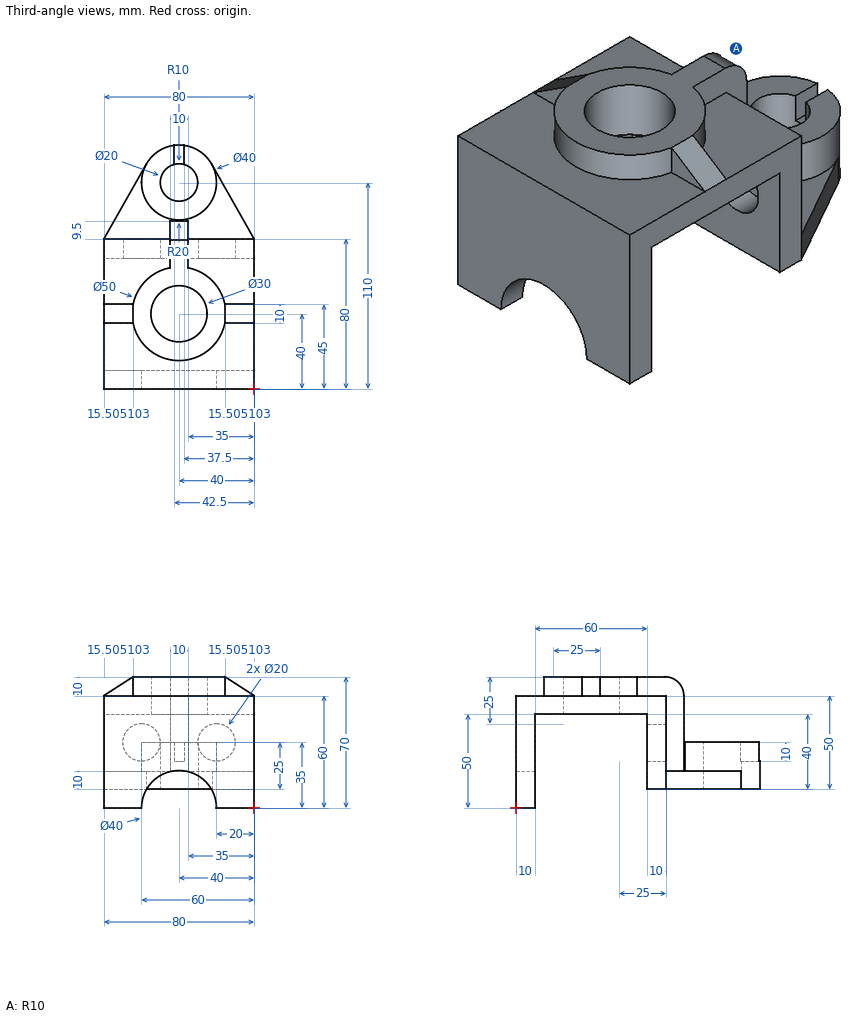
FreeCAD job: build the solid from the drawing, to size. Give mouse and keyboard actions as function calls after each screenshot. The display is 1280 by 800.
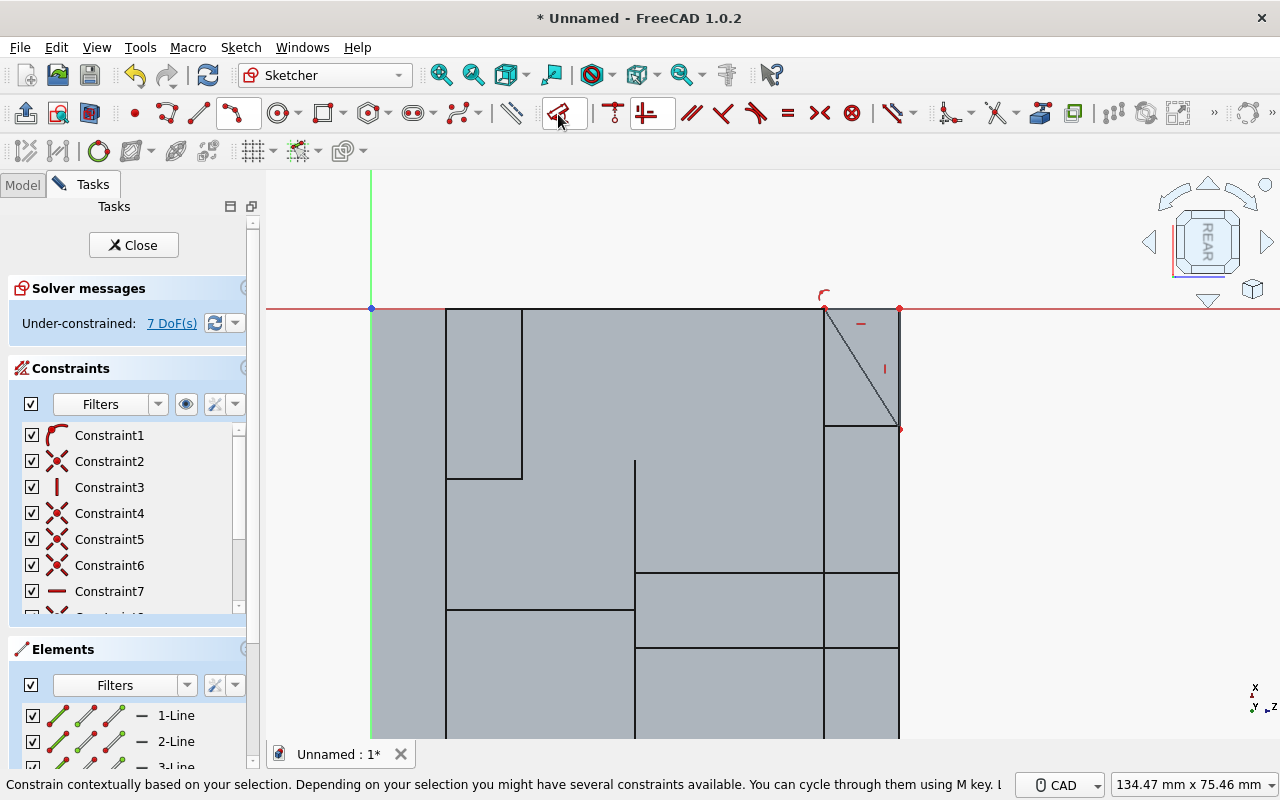
click(877, 309)
click(862, 275)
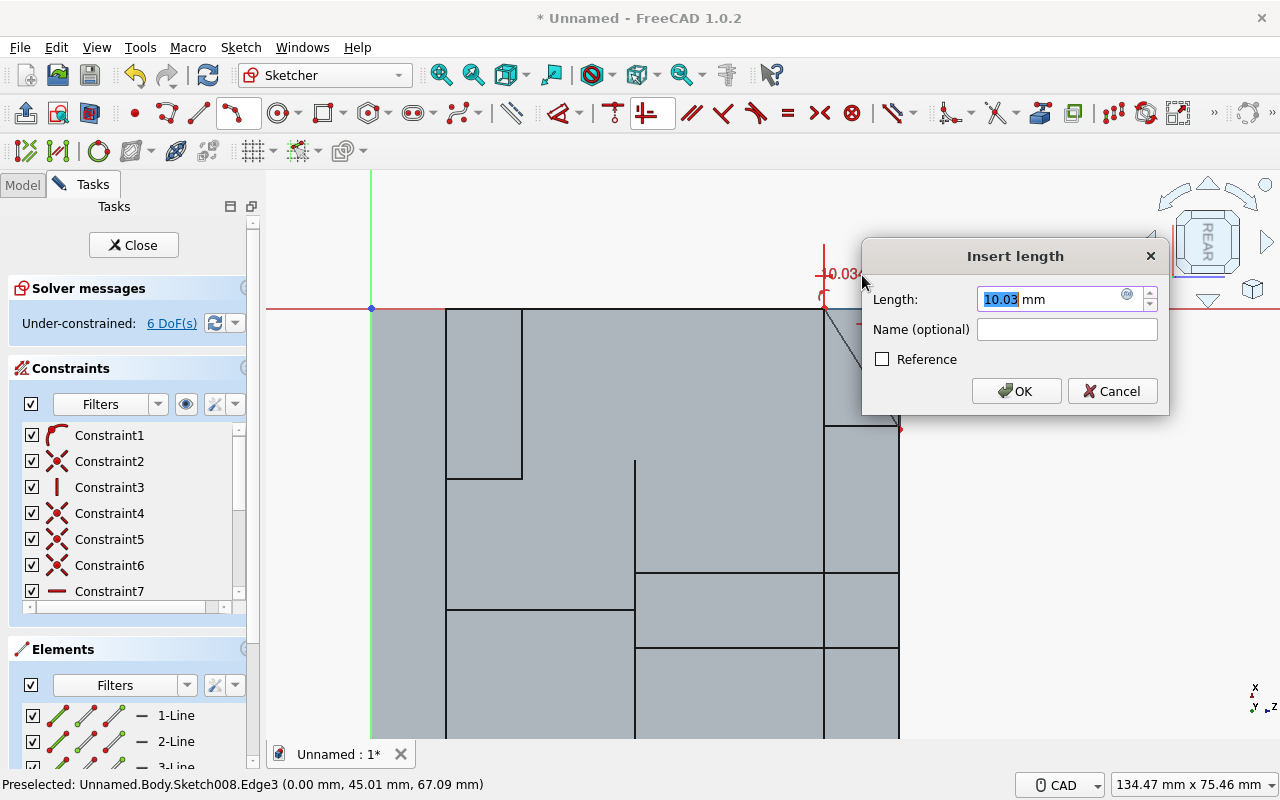
text(10)
key(Return)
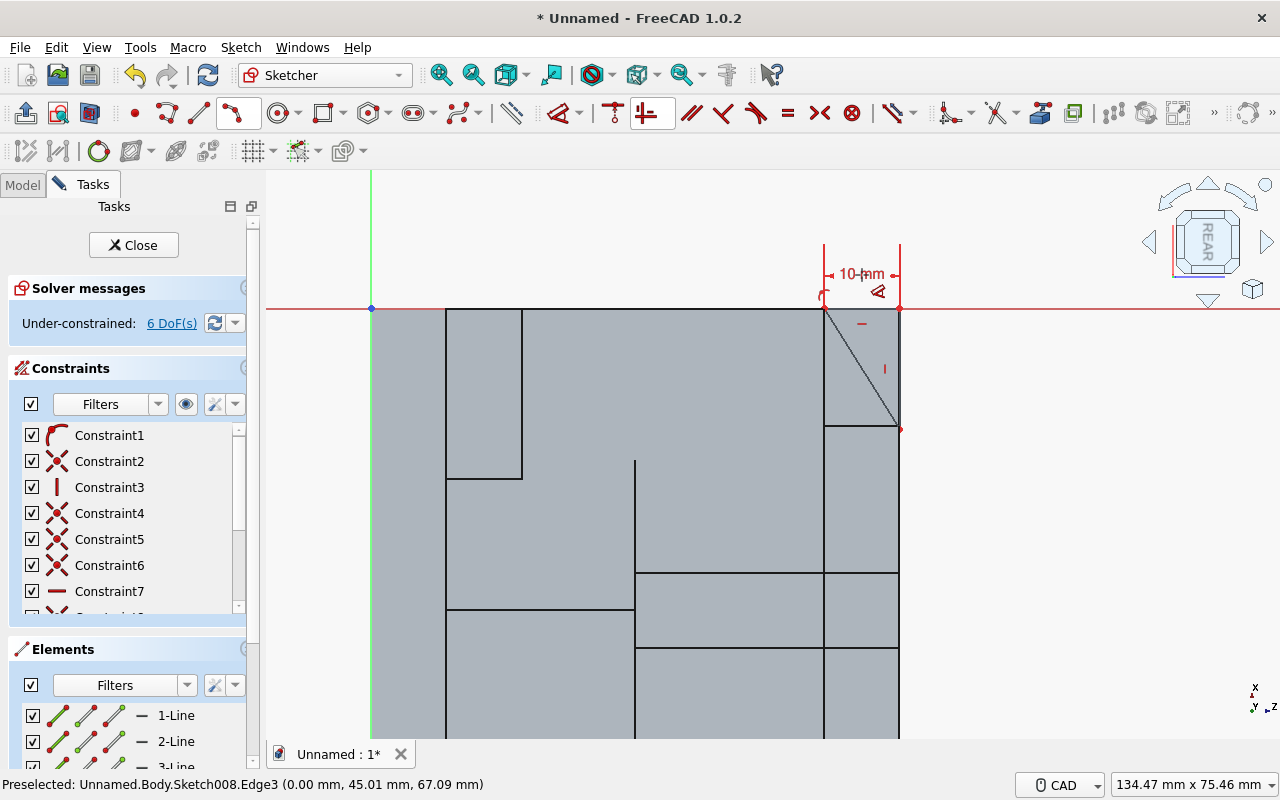
scroll(789, 265, down, 3)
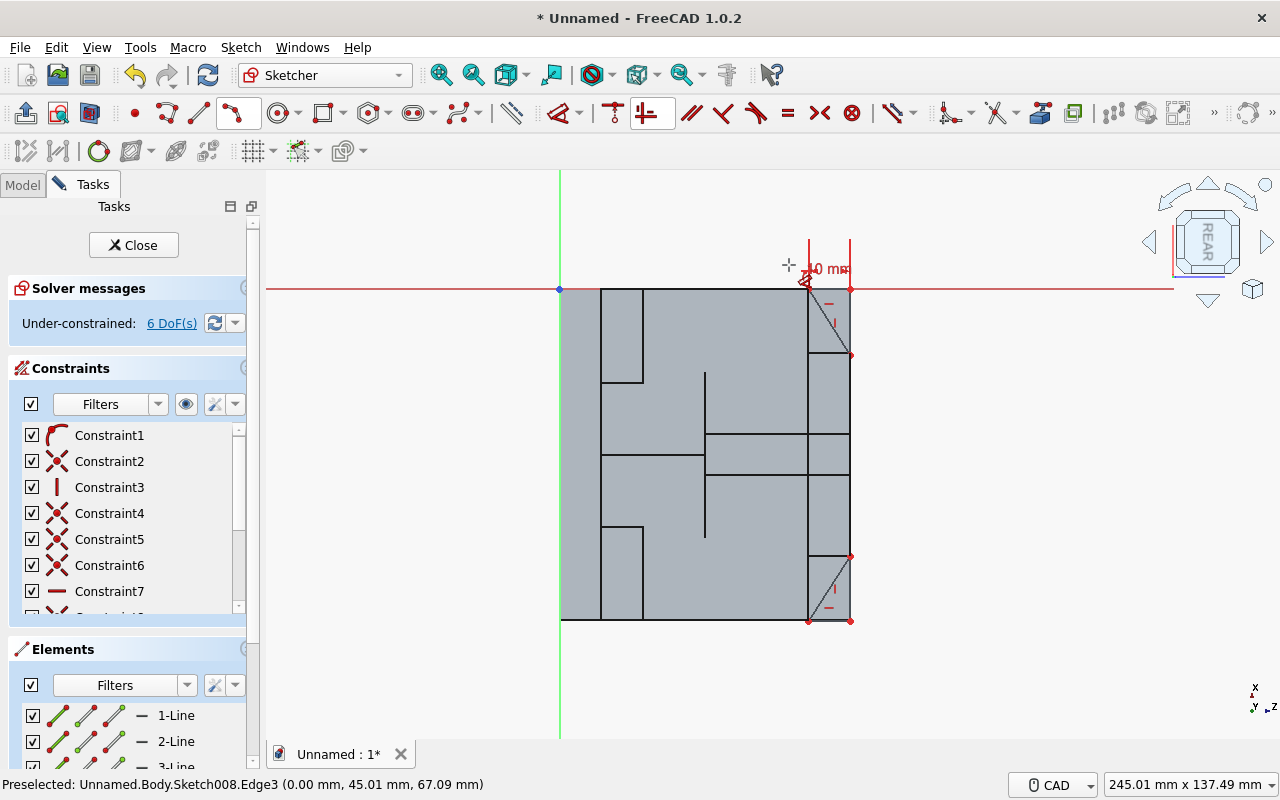
scroll(821, 621, up, 2)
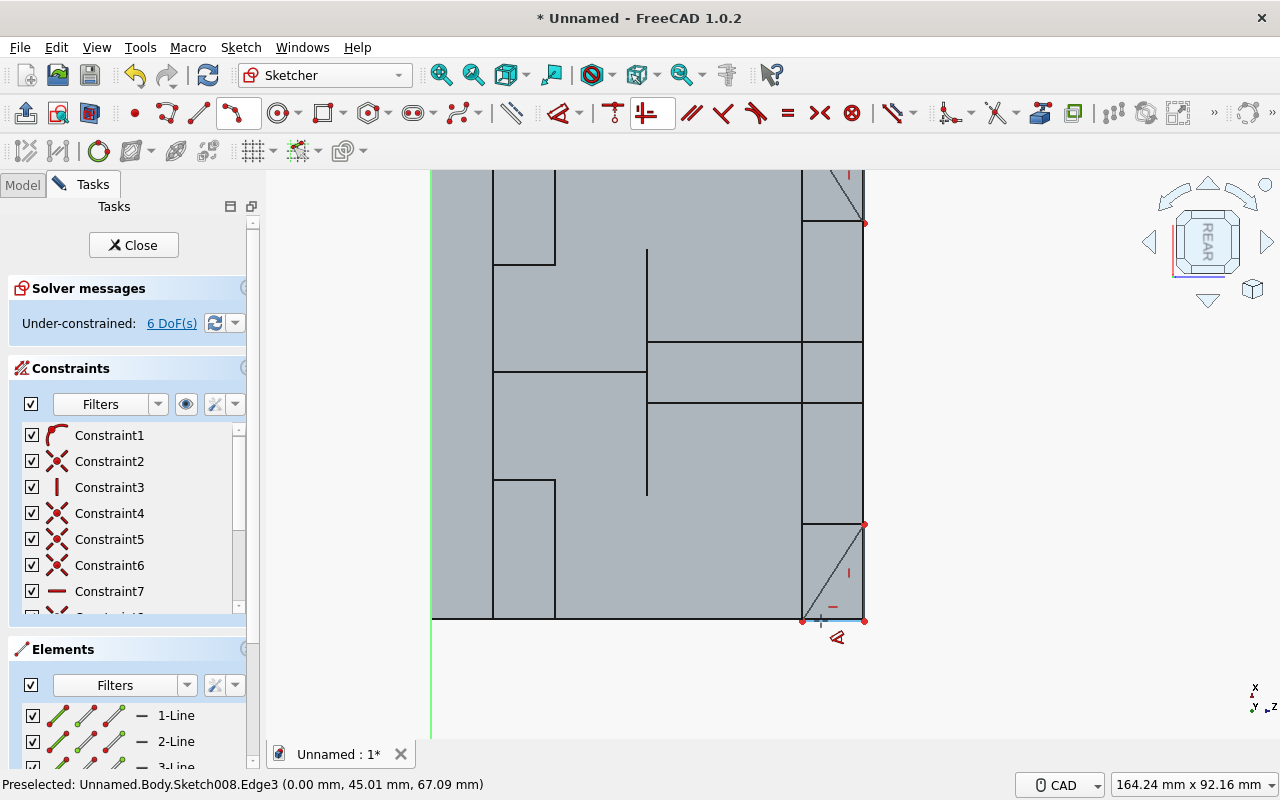
click(821, 621)
click(833, 655)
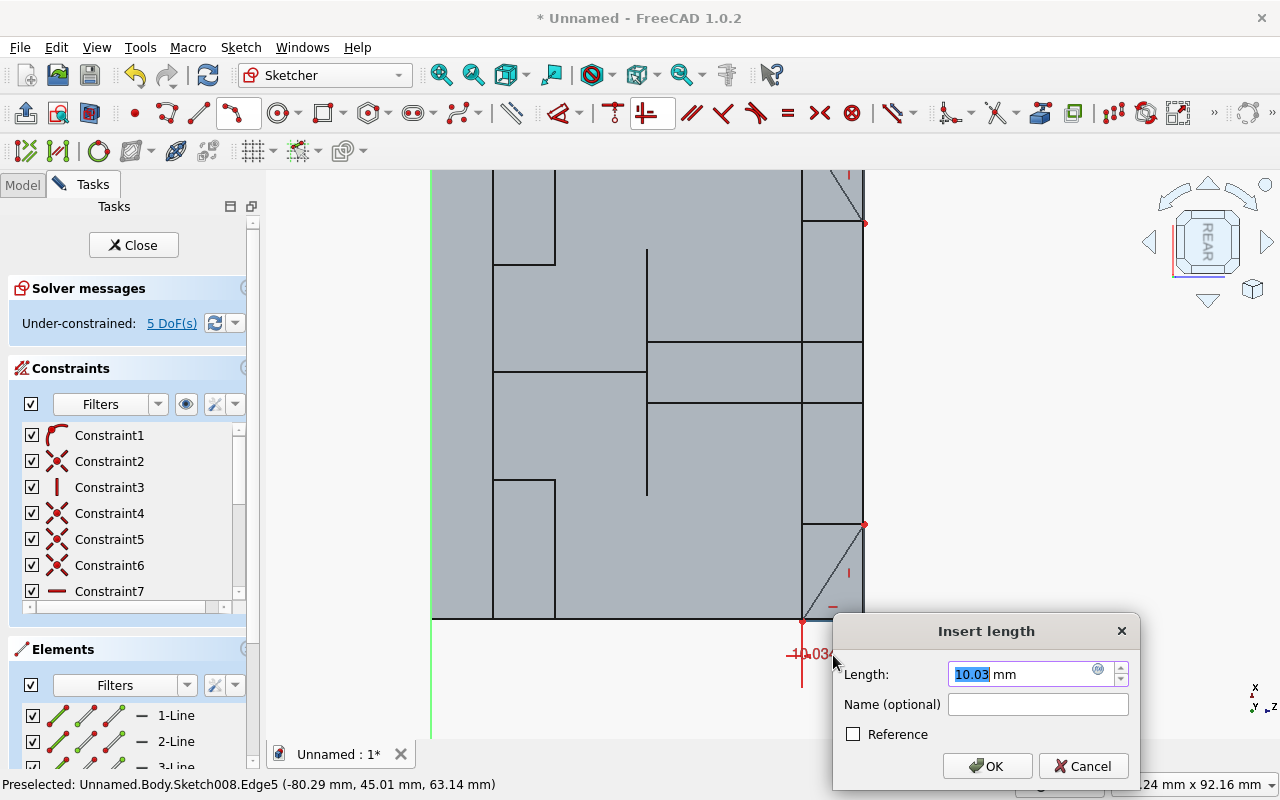
text(10)
key(Return)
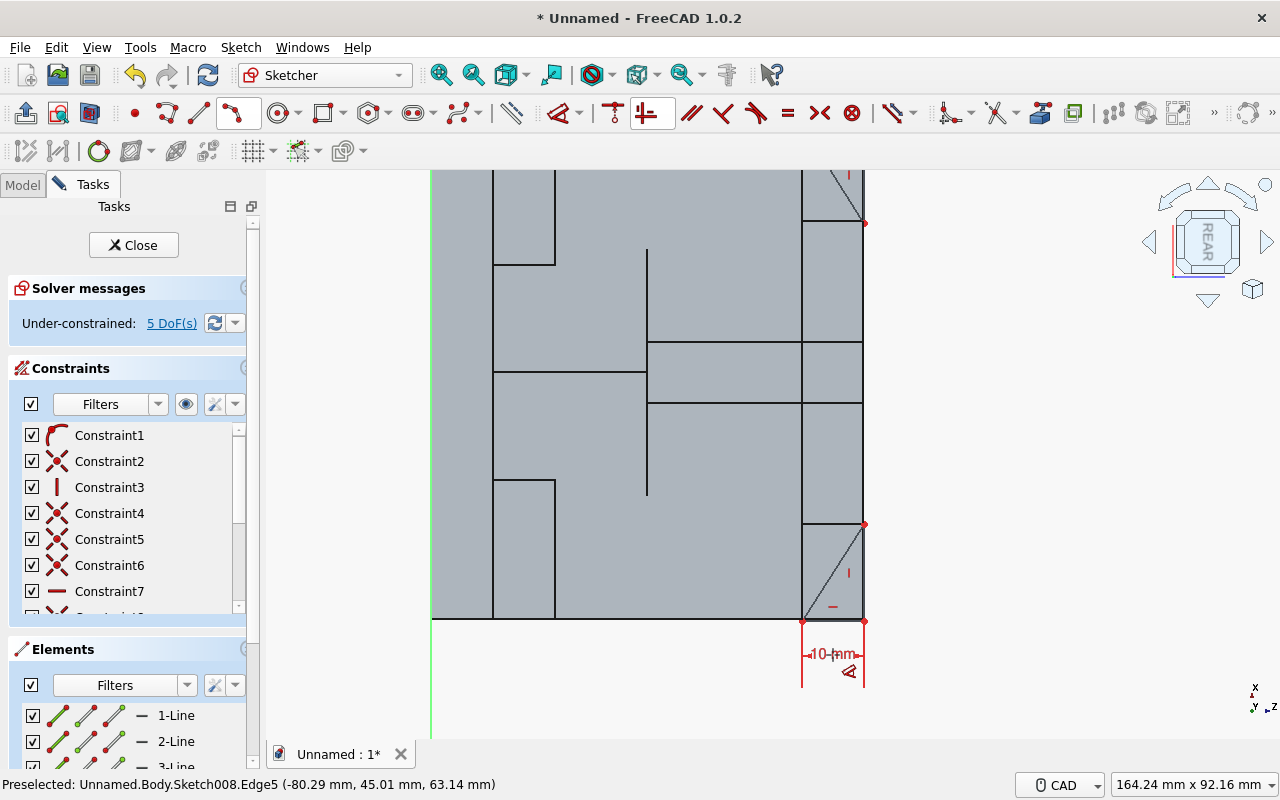
scroll(821, 621, down, 2)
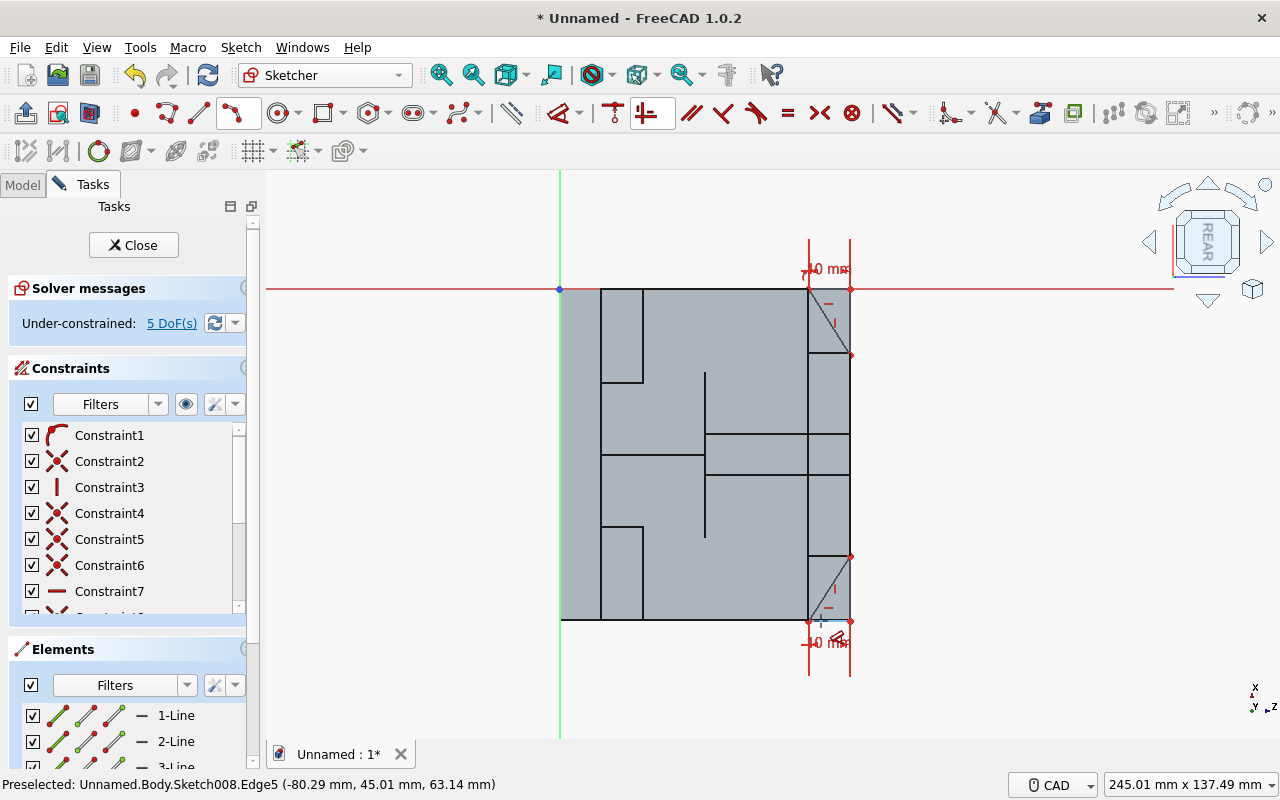
click(809, 289)
click(684, 255)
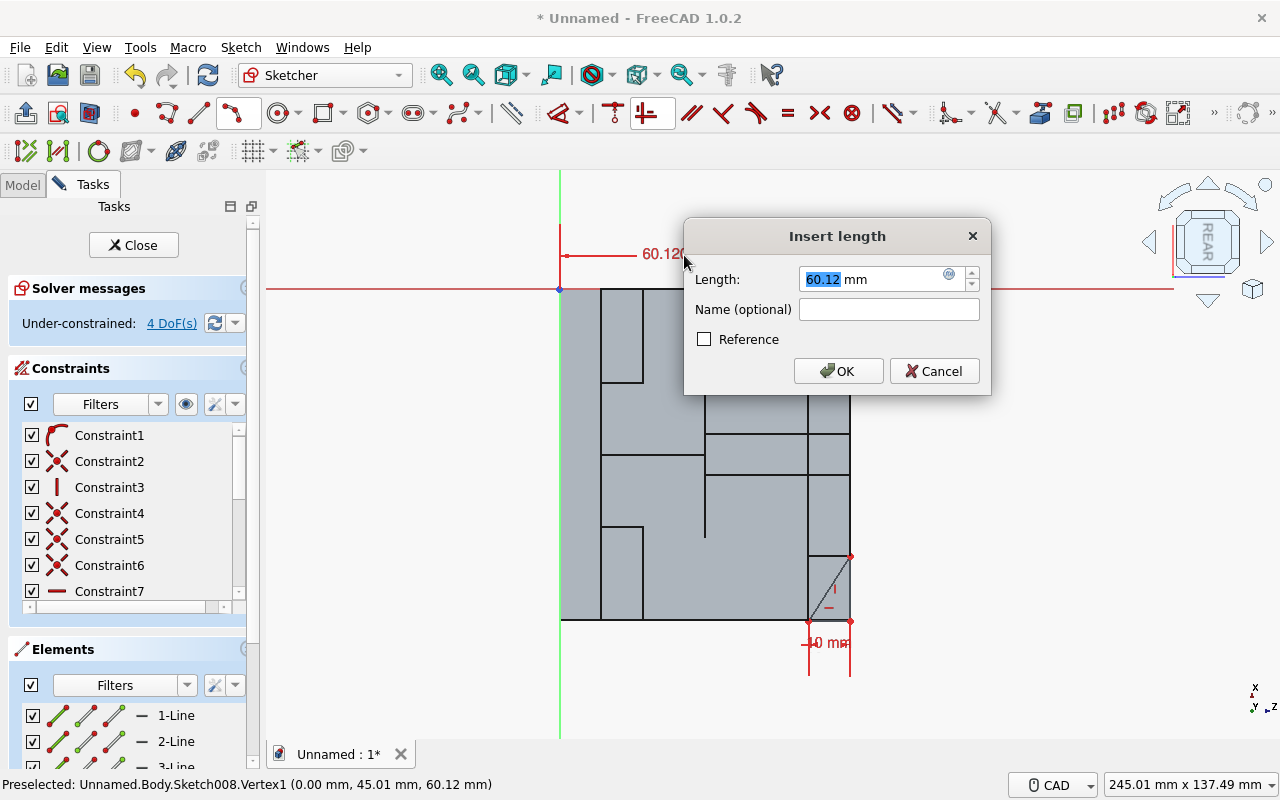
text(60)
key(Return)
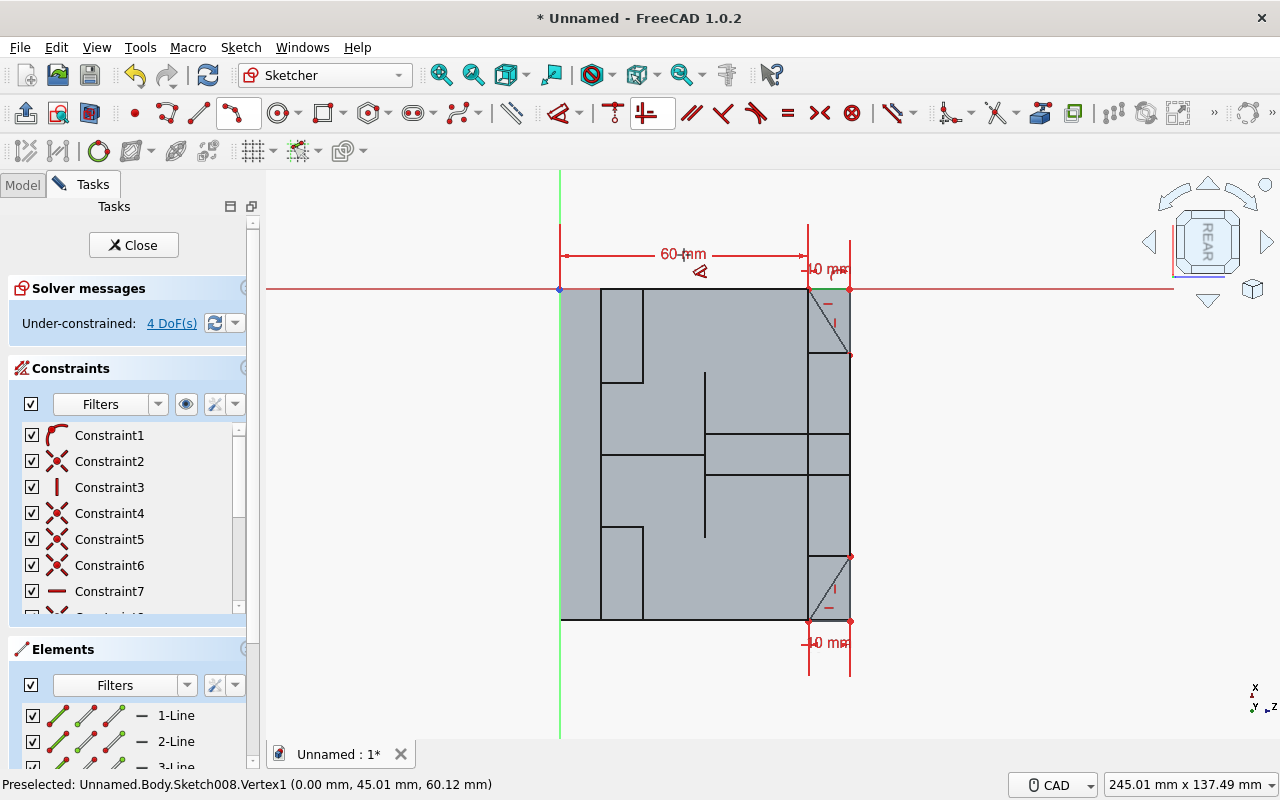
click(850, 557)
click(603, 255)